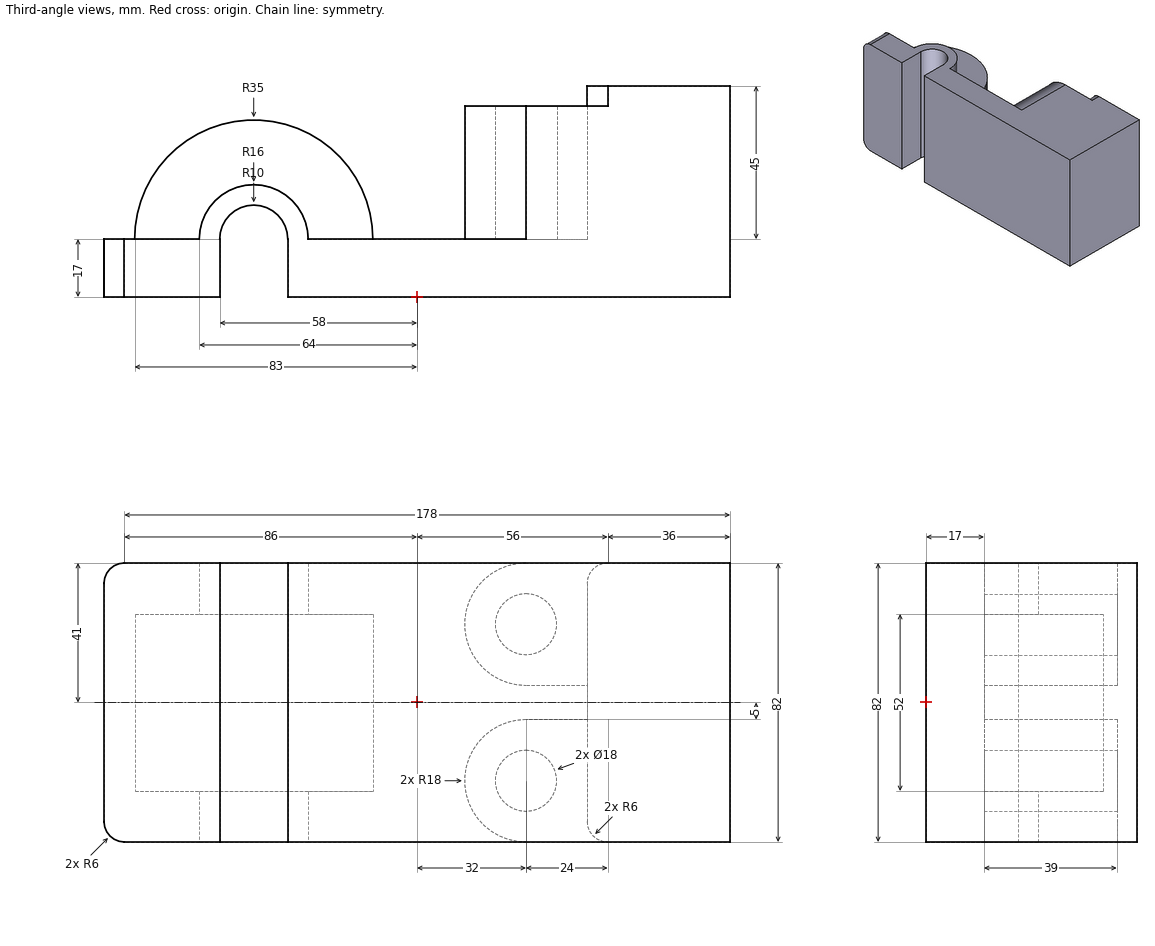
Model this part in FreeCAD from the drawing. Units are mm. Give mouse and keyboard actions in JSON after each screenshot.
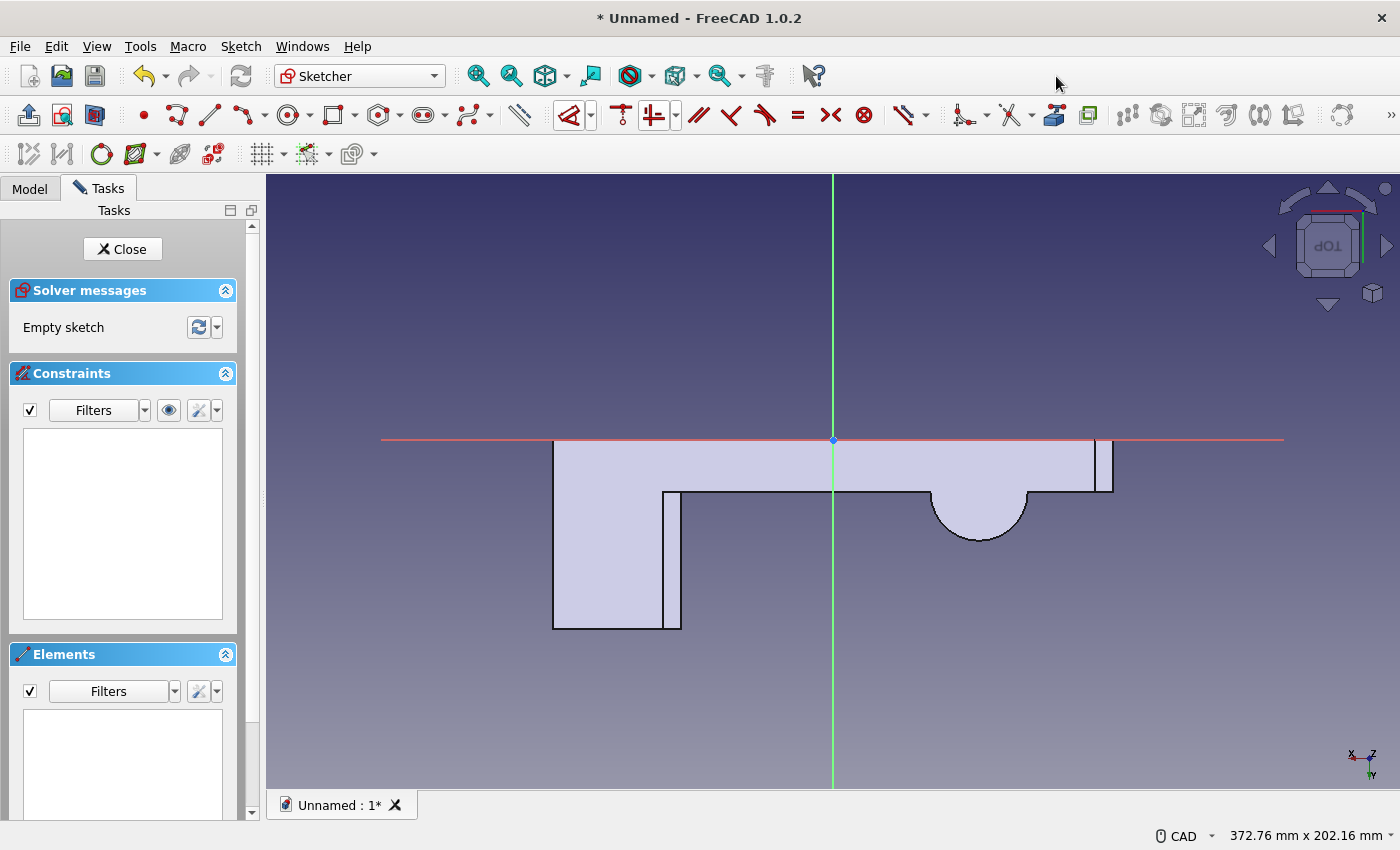
{"action": "scroll", "coordinate": [973, 482], "scroll_direction": "up", "scroll_amount": 7}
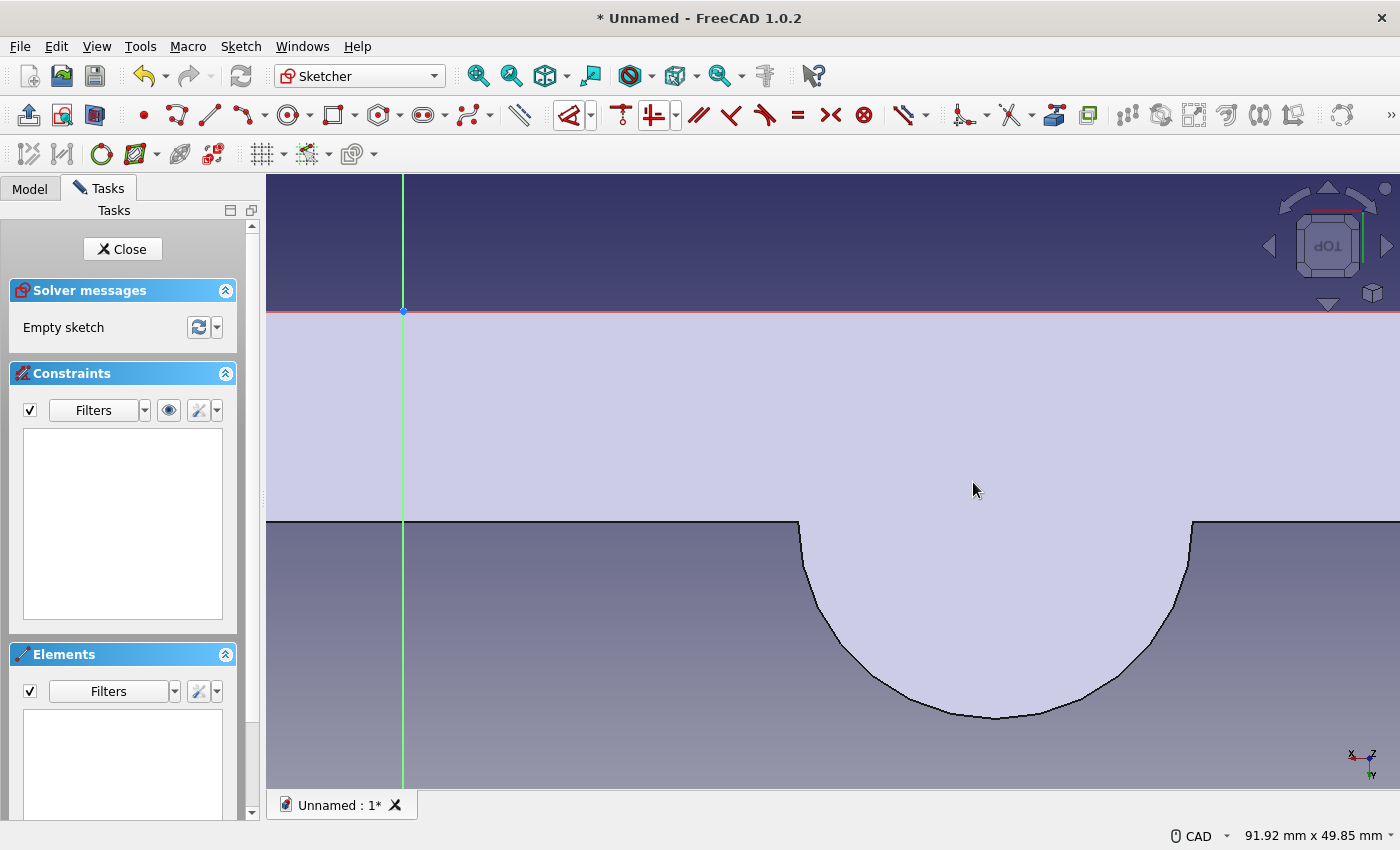
{"action": "left_click", "coordinate": [177, 116]}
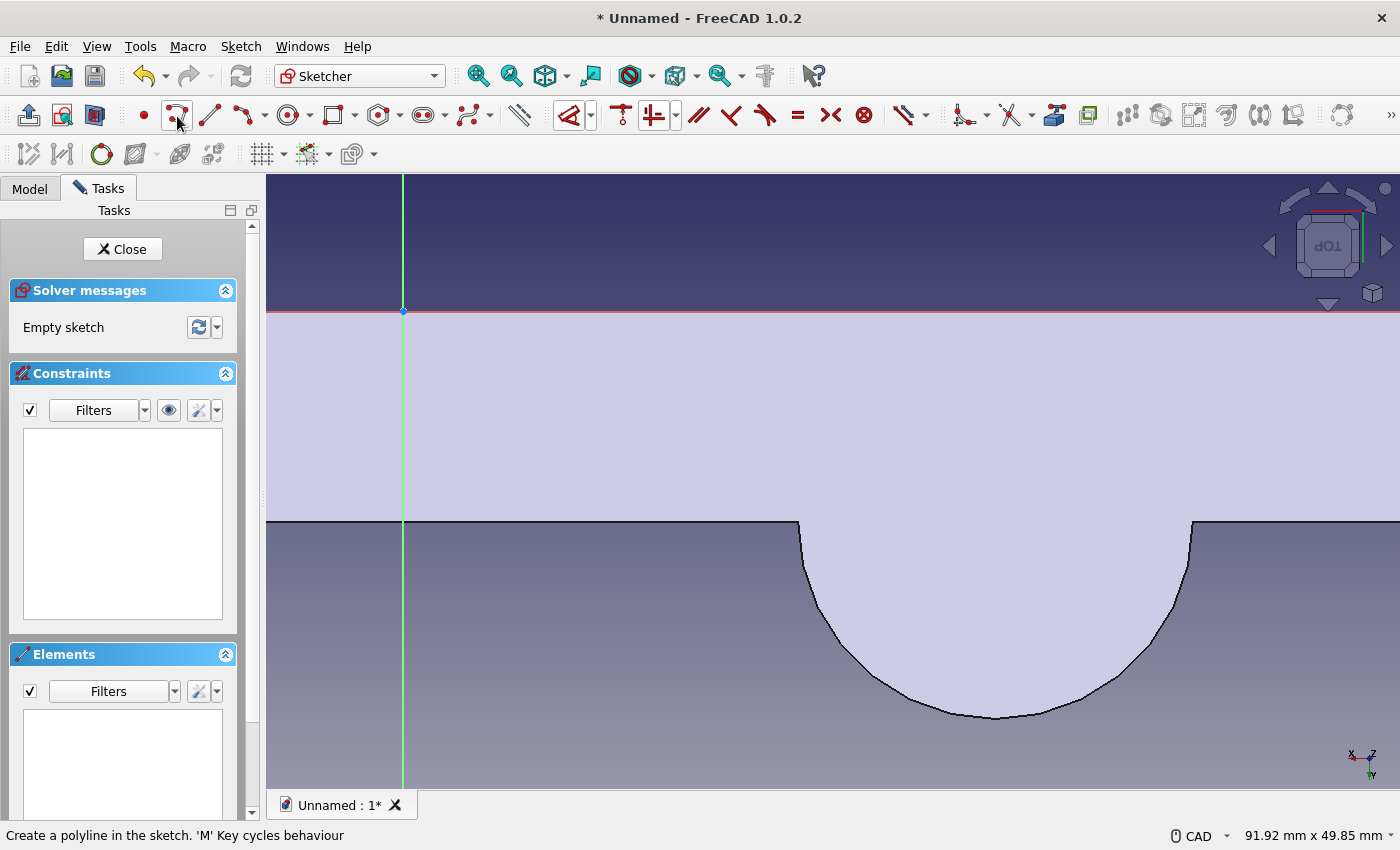
{"action": "left_click", "coordinate": [1119, 522]}
{"action": "left_click", "coordinate": [1119, 312]}
{"action": "left_click", "coordinate": [872, 321]}
{"action": "left_click", "coordinate": [872, 522]}
{"action": "right_click", "coordinate": [872, 522]}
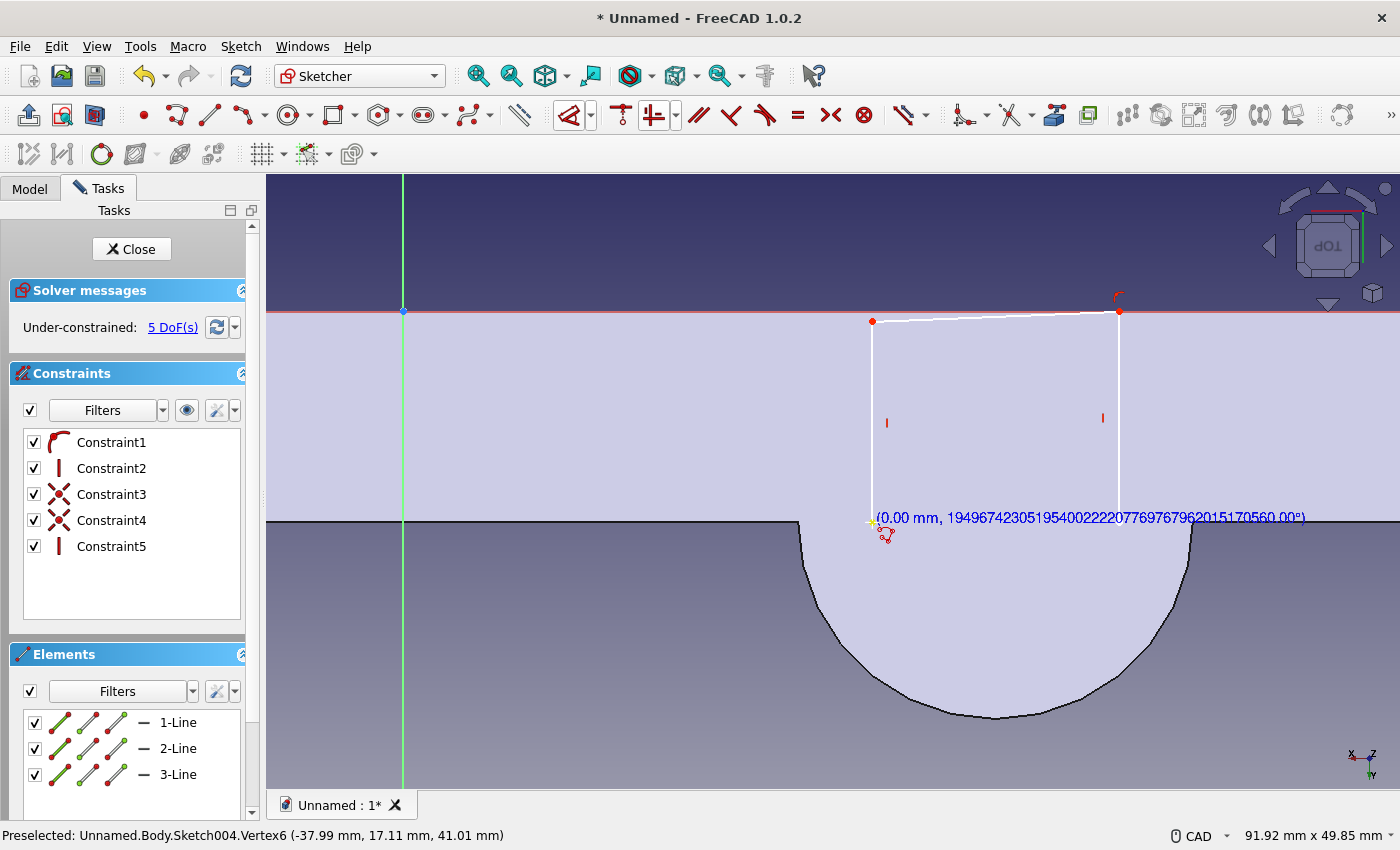
{"action": "left_click", "coordinate": [242, 116]}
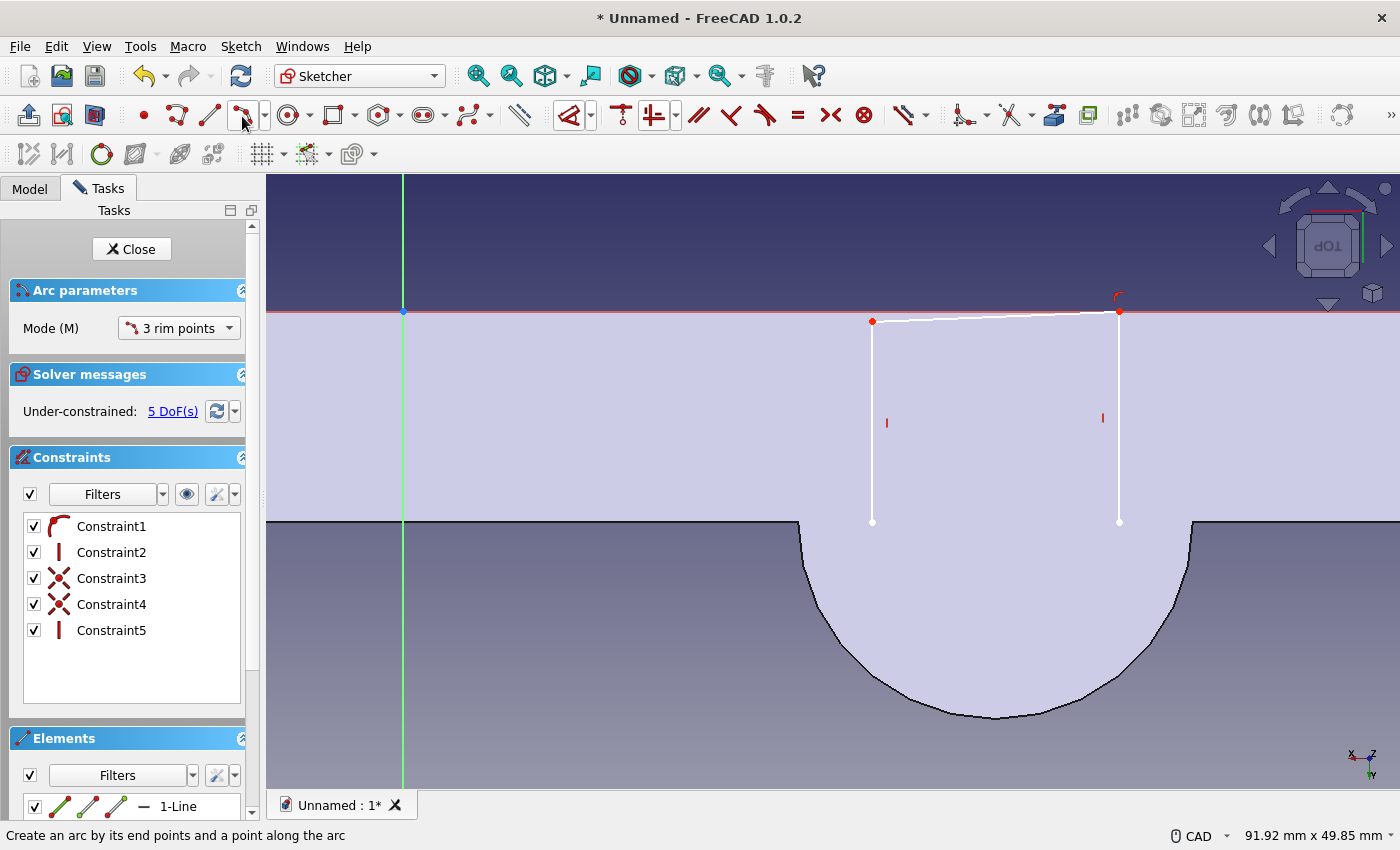
{"action": "left_click", "coordinate": [872, 523]}
{"action": "left_click", "coordinate": [1119, 523]}
{"action": "left_click", "coordinate": [996, 645]}
{"action": "key", "text": "Escape"}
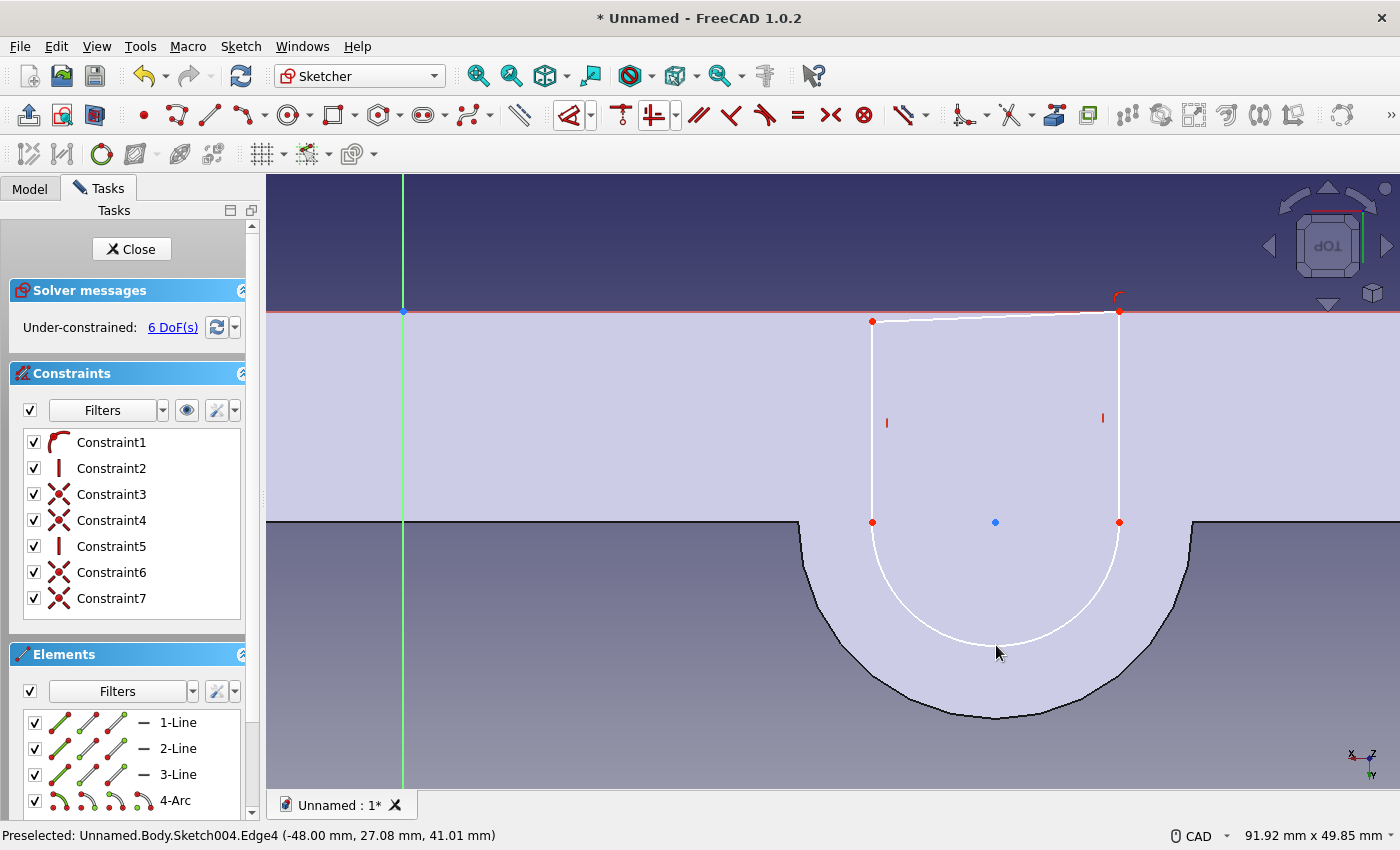
{"action": "left_click", "coordinate": [1119, 460]}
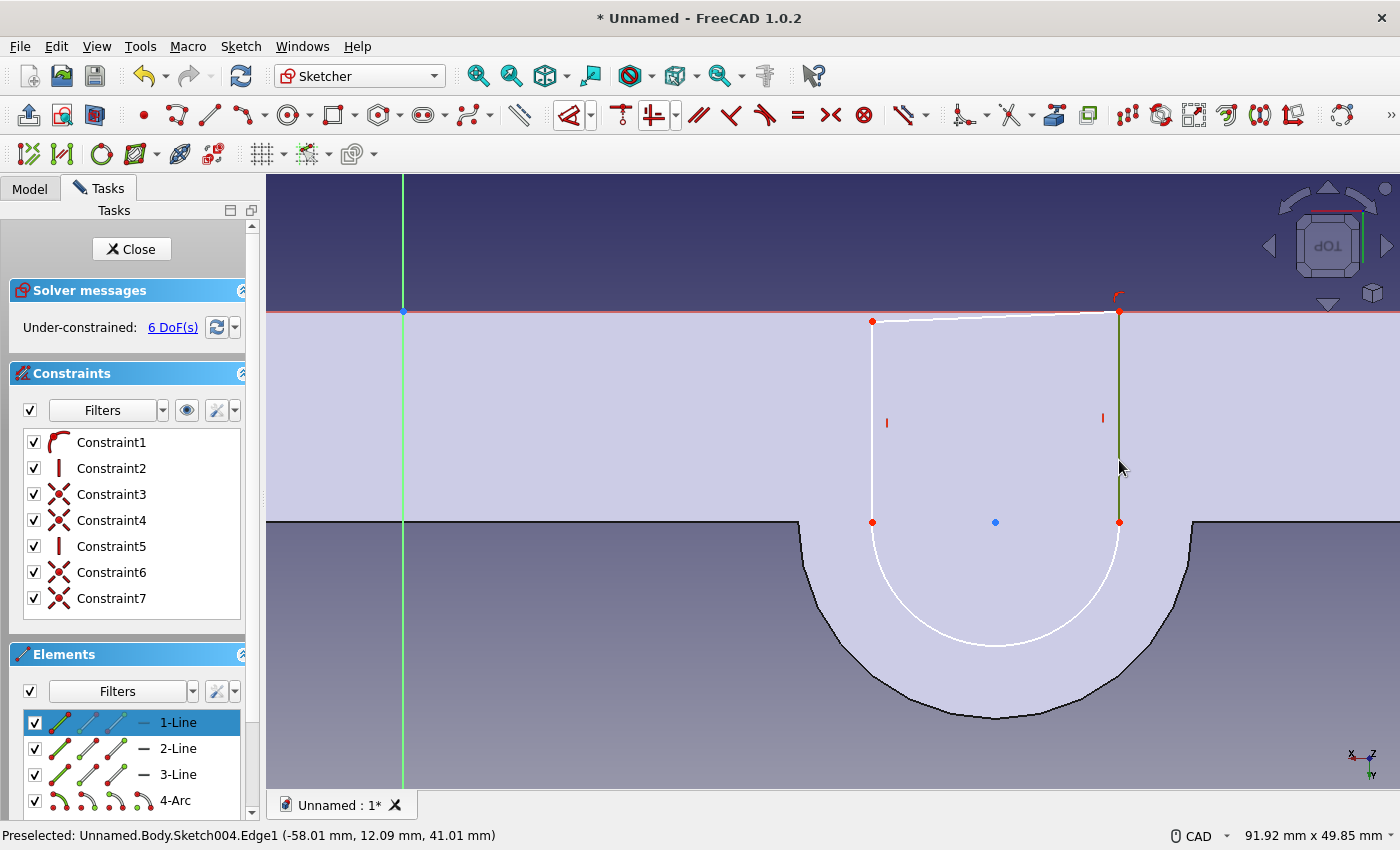
{"action": "left_click", "coordinate": [923, 623]}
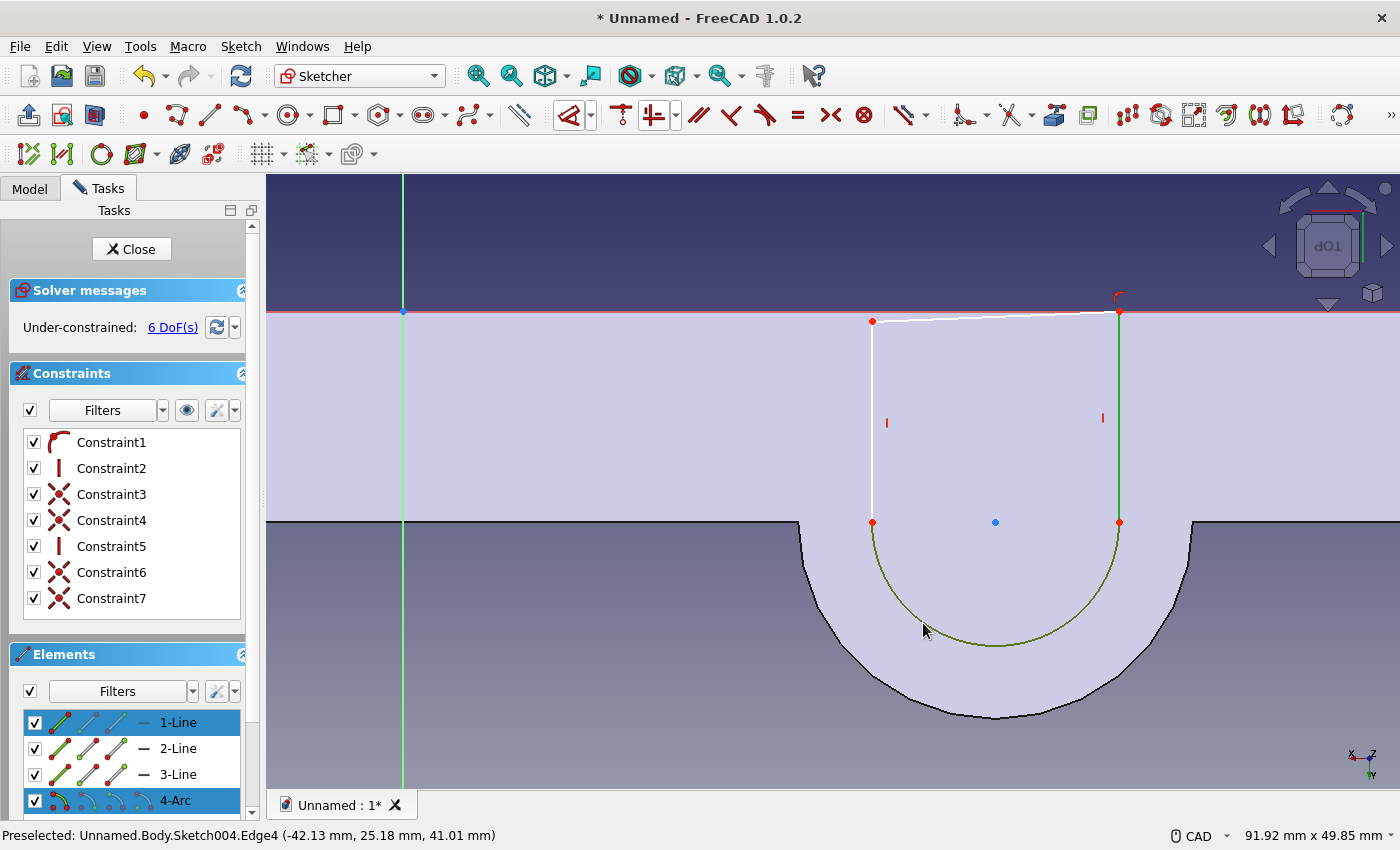
{"action": "left_click", "coordinate": [765, 116]}